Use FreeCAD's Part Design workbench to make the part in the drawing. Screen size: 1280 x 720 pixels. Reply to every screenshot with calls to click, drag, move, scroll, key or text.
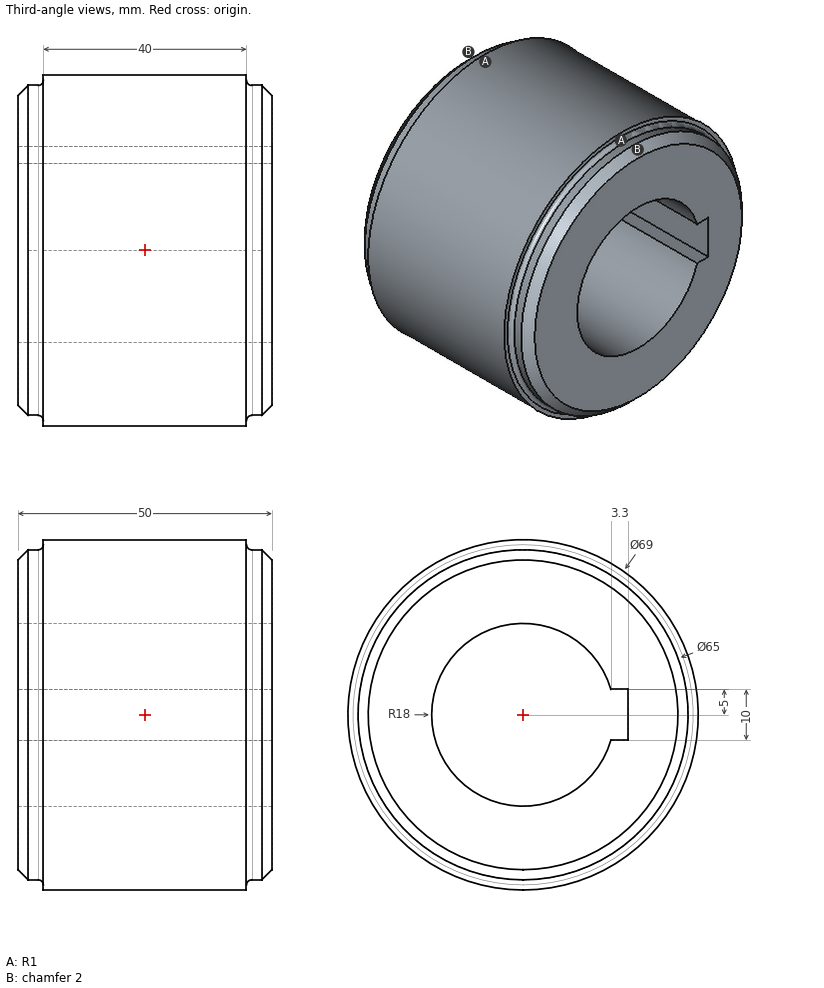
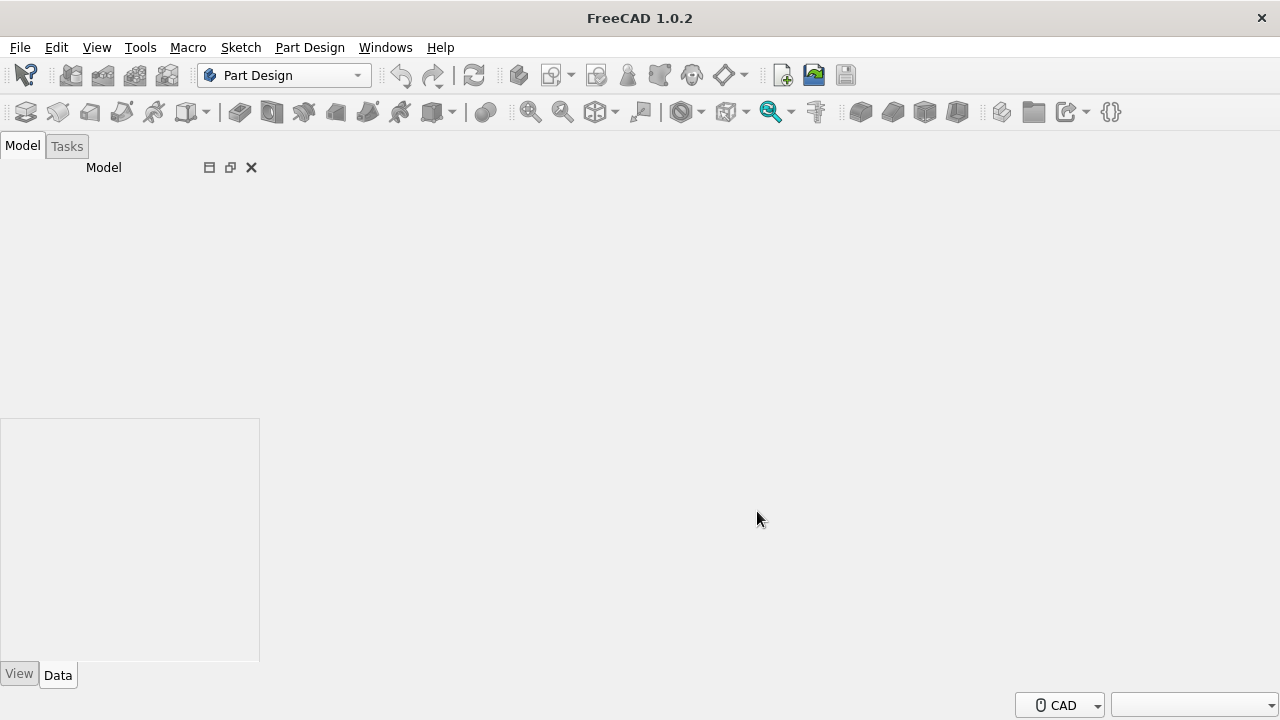
key(ctrl+n)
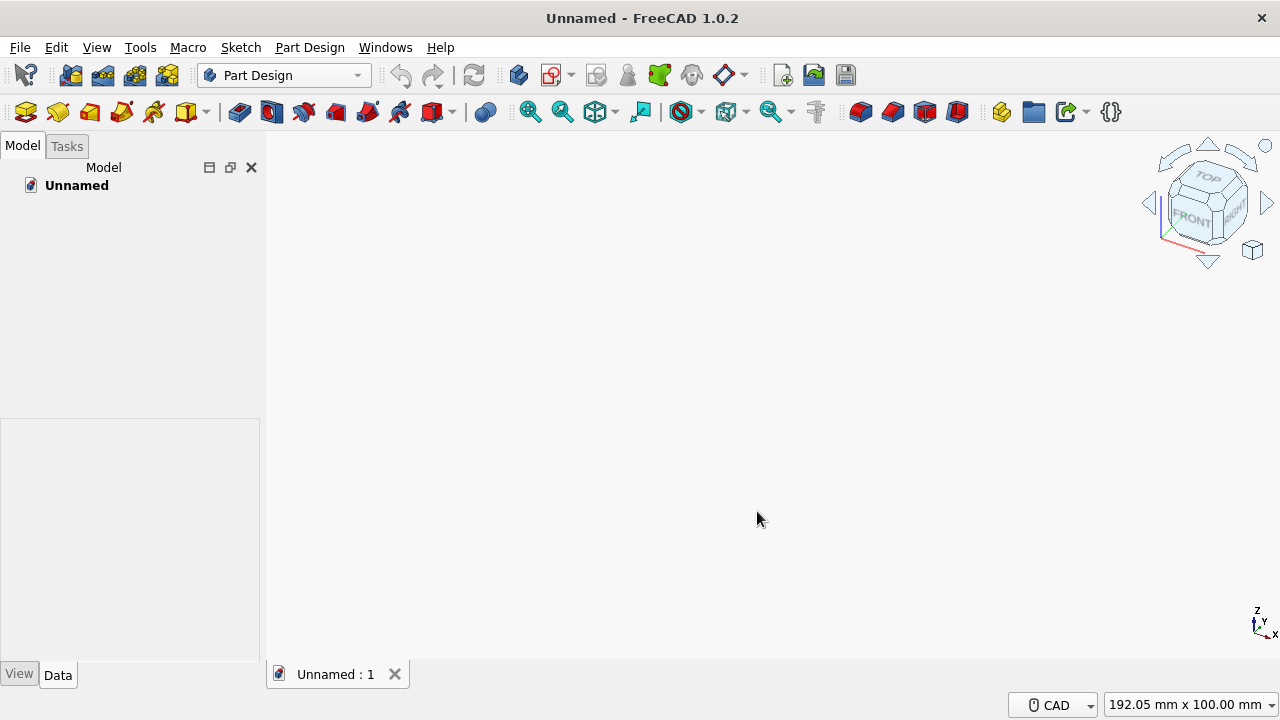
click(552, 76)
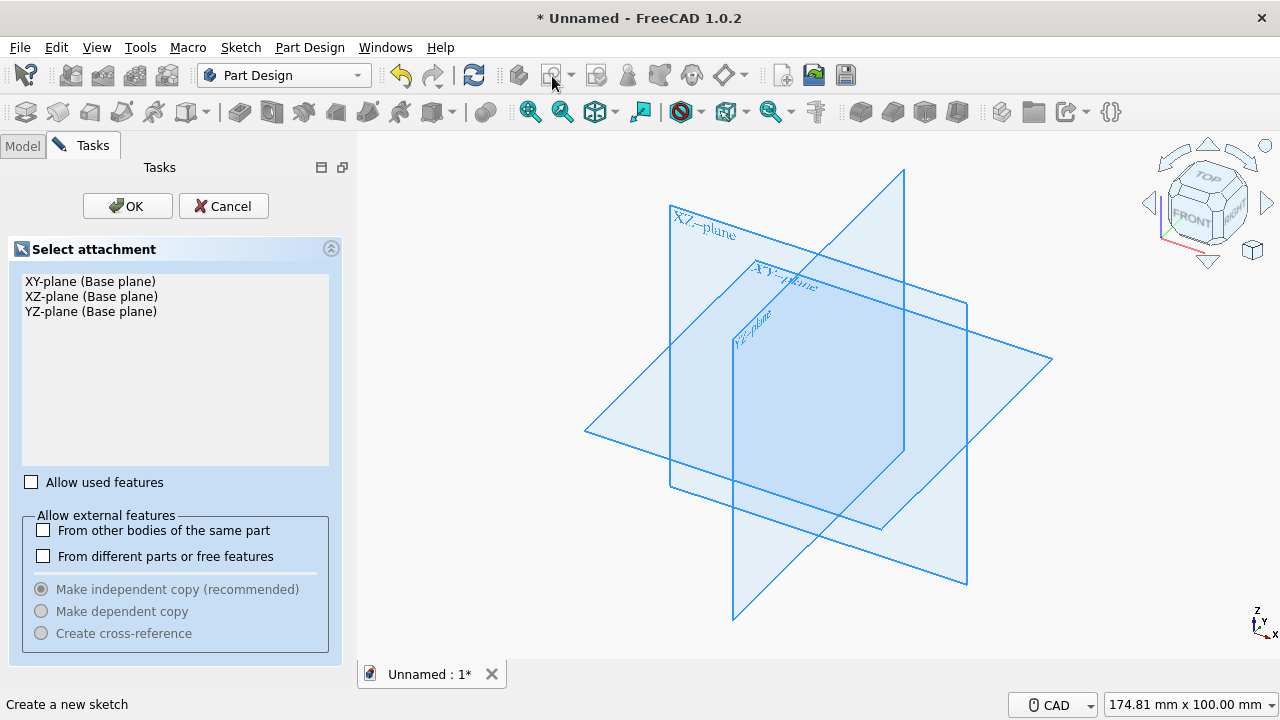
click(82, 312)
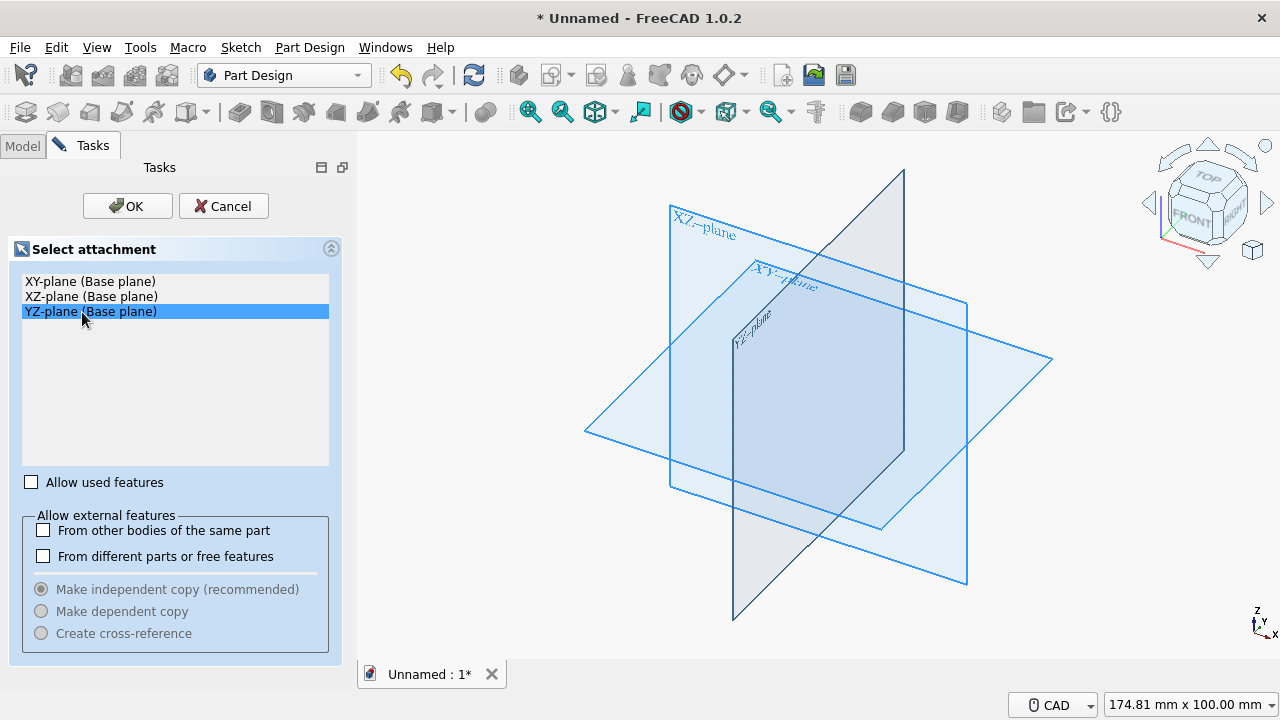
click(128, 206)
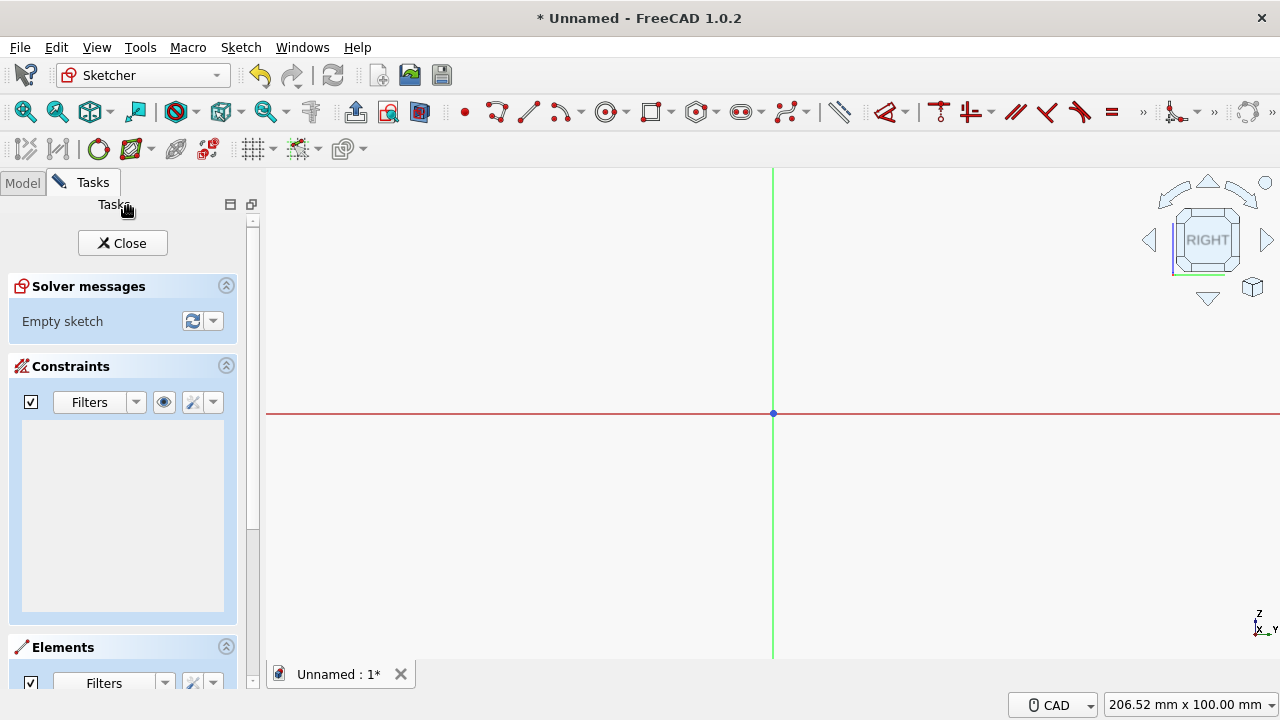
key(g)
key(m)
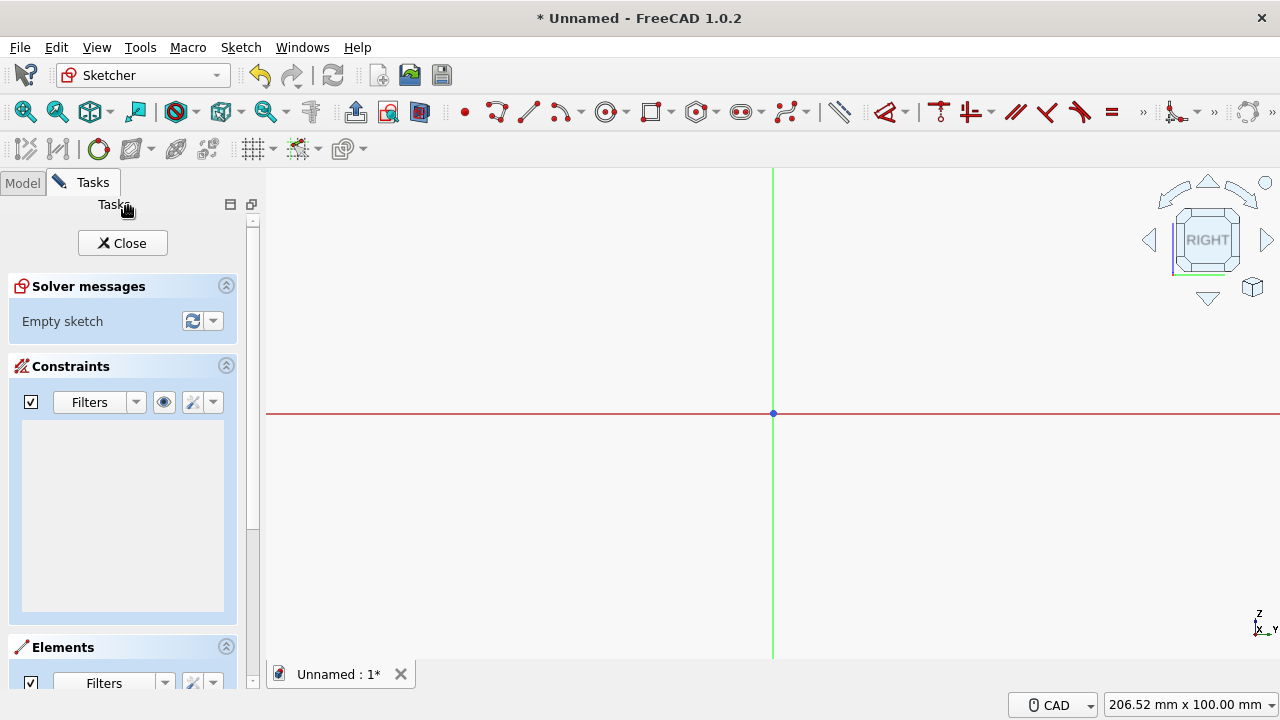
click(858, 389)
click(874, 389)
click(874, 438)
click(858, 438)
right_click(858, 438)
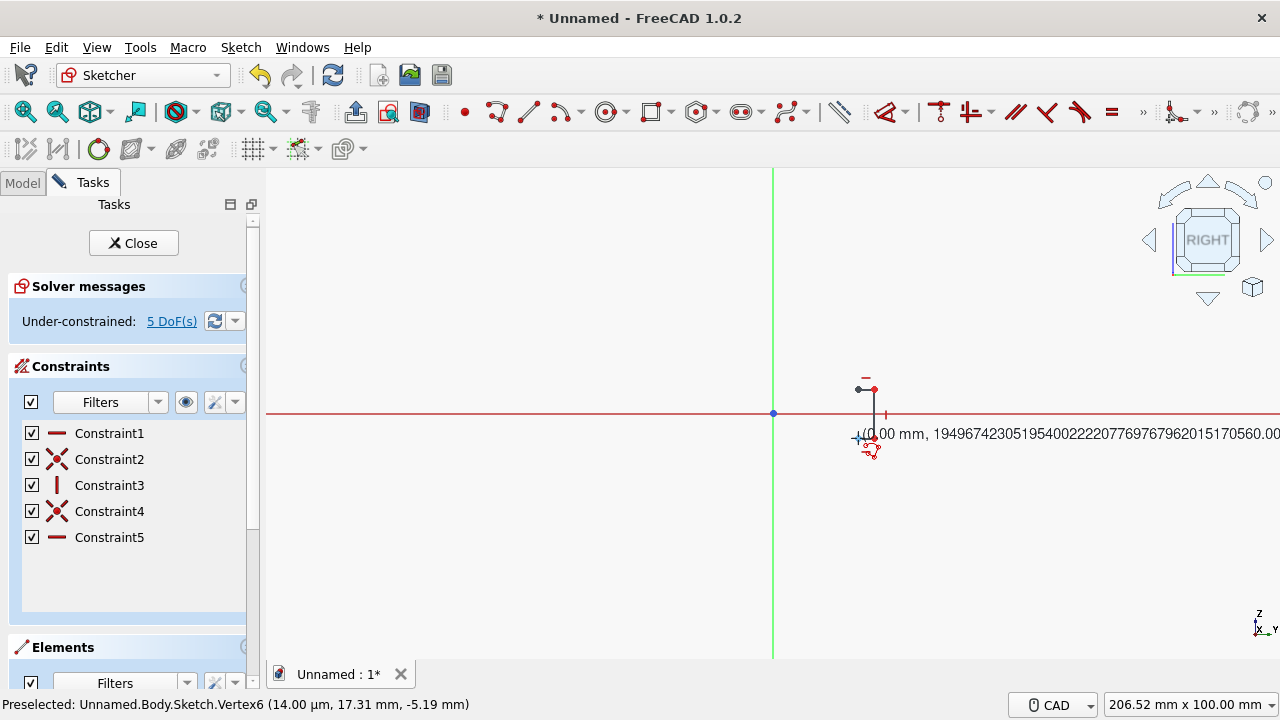
key(g)
key(3)
key(a)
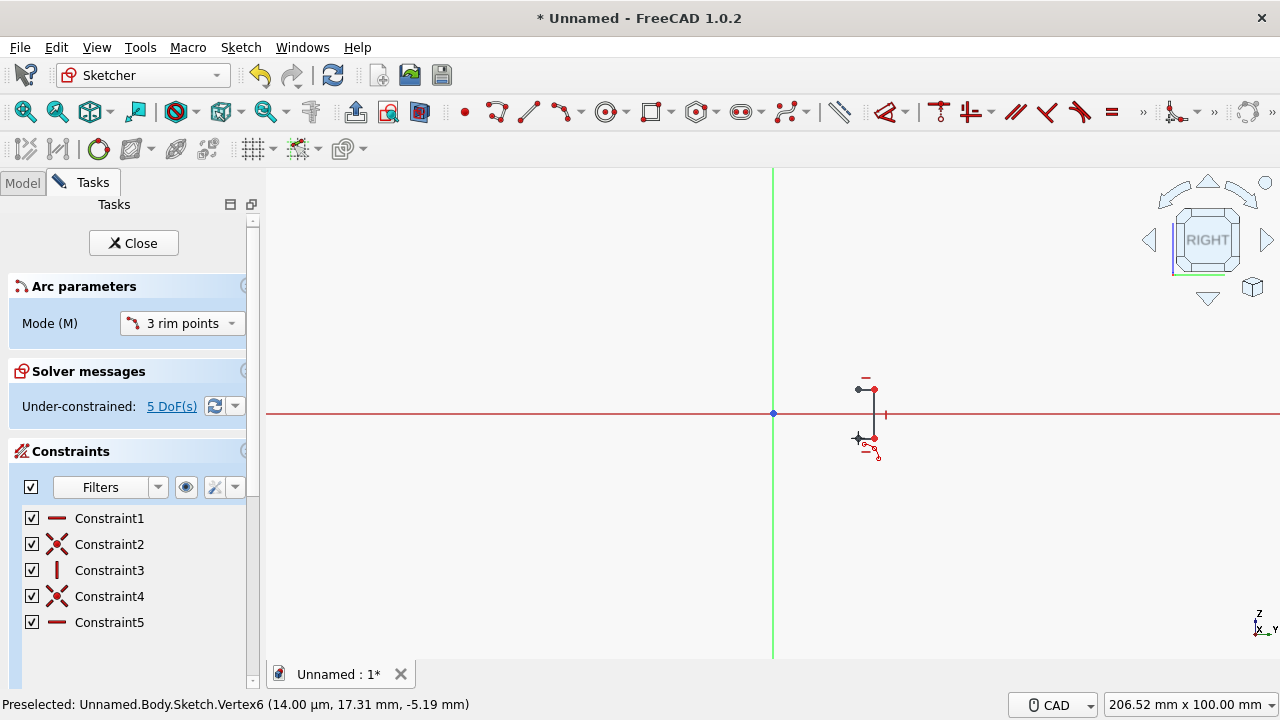
scroll(858, 438, up, 4)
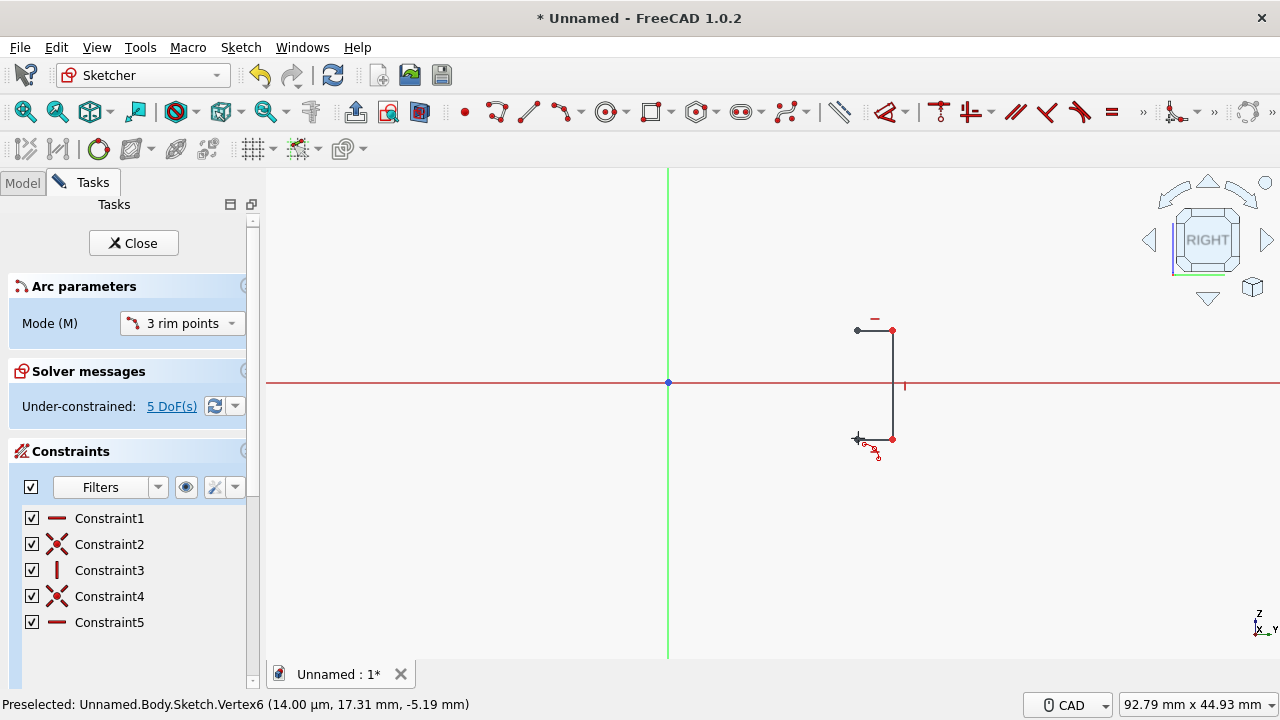
click(857, 440)
click(857, 330)
click(503, 276)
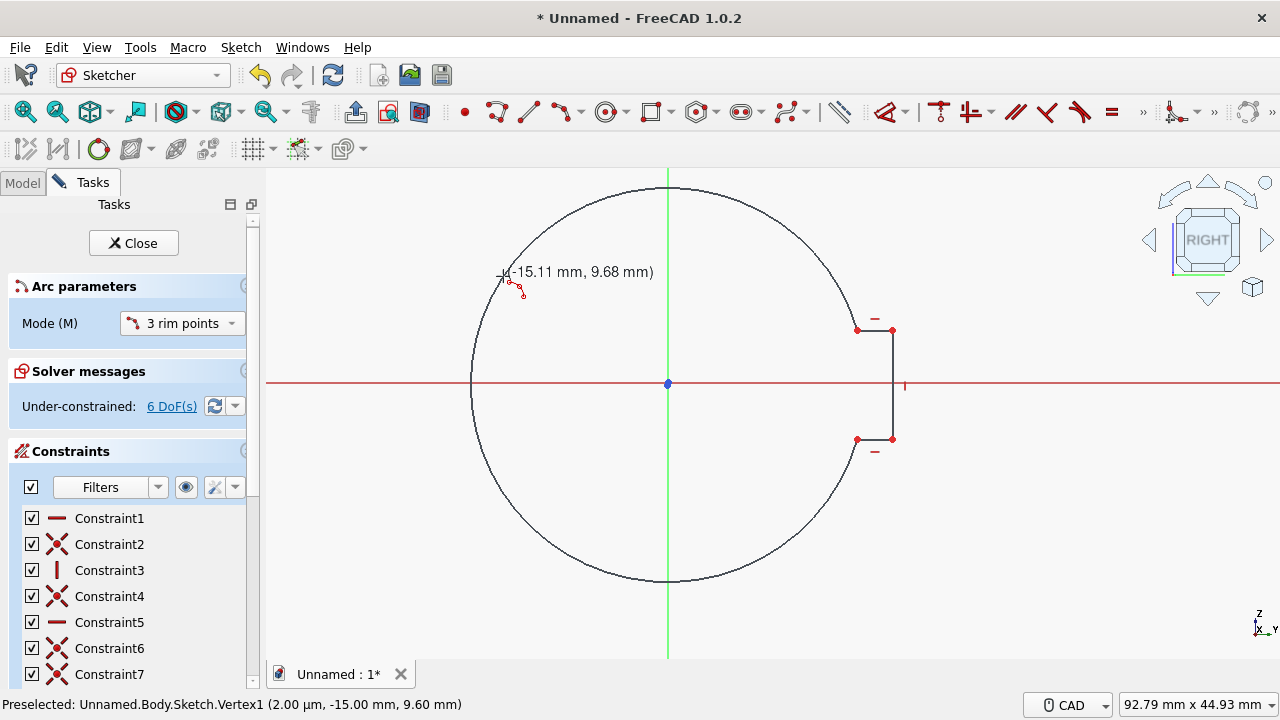
click(606, 112)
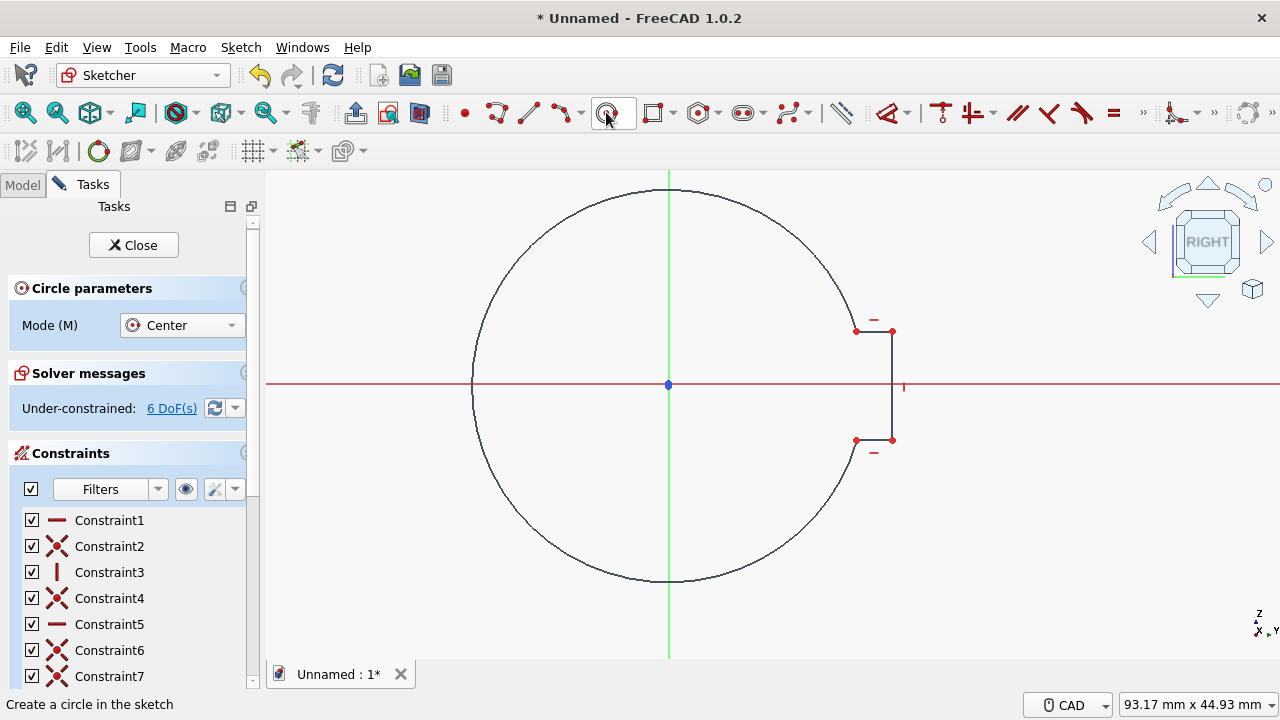
click(669, 384)